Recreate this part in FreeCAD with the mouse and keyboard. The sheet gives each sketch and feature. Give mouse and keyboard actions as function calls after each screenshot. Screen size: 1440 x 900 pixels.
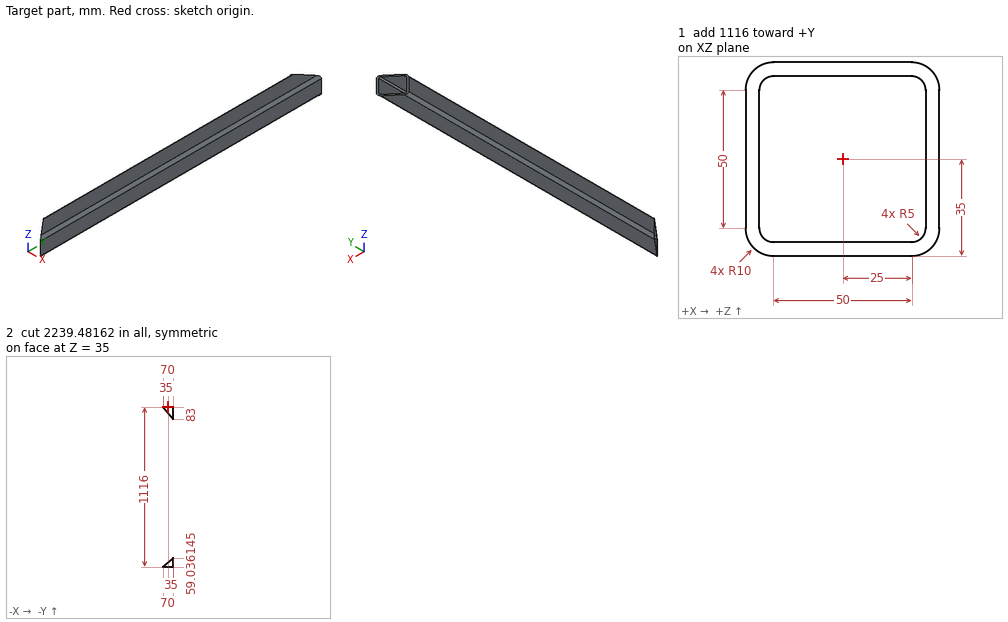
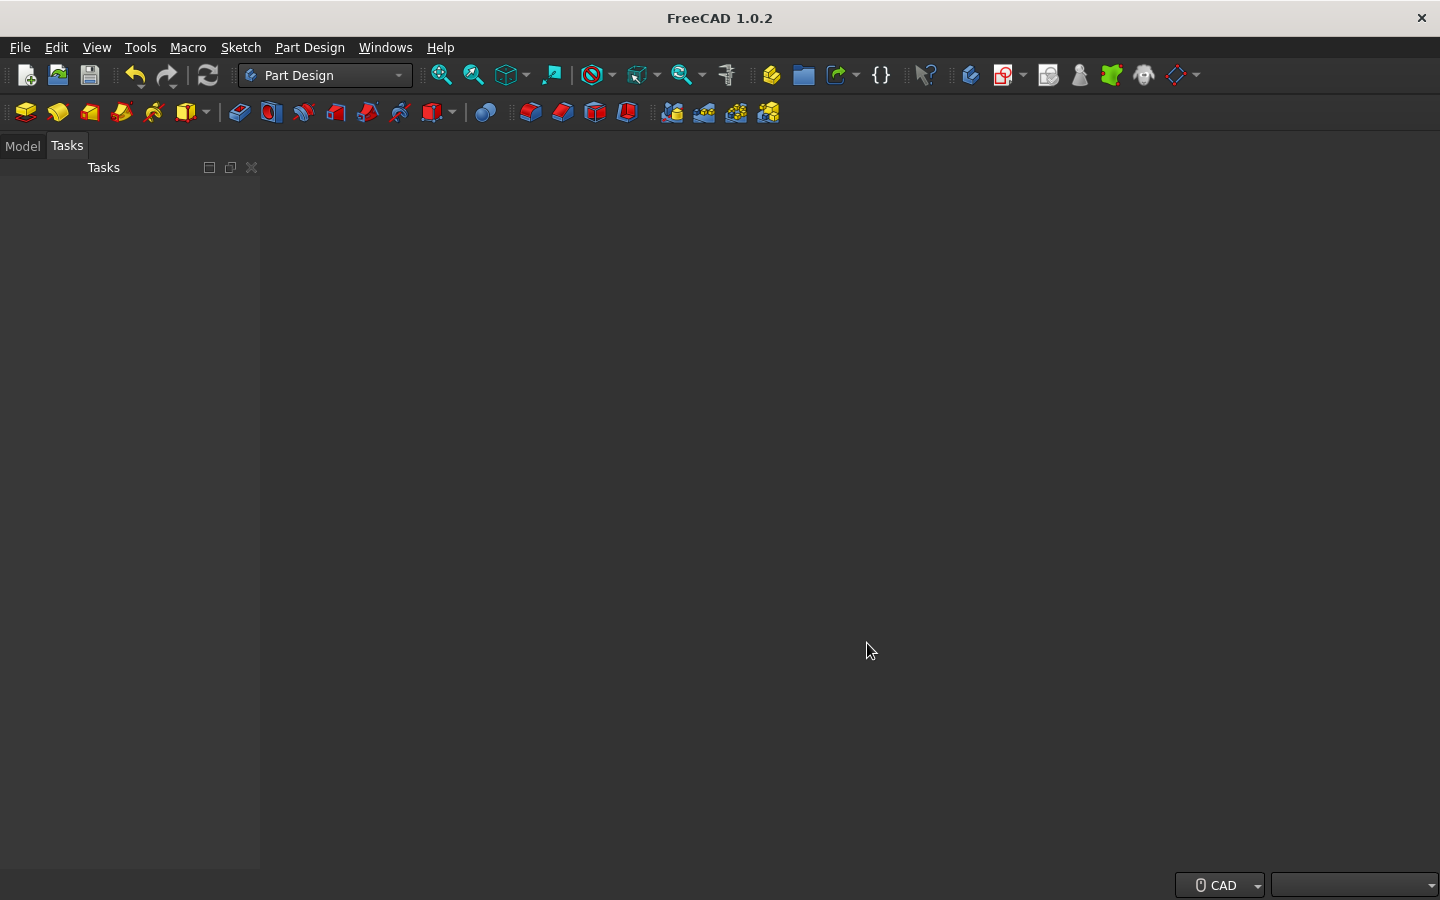
click(26, 76)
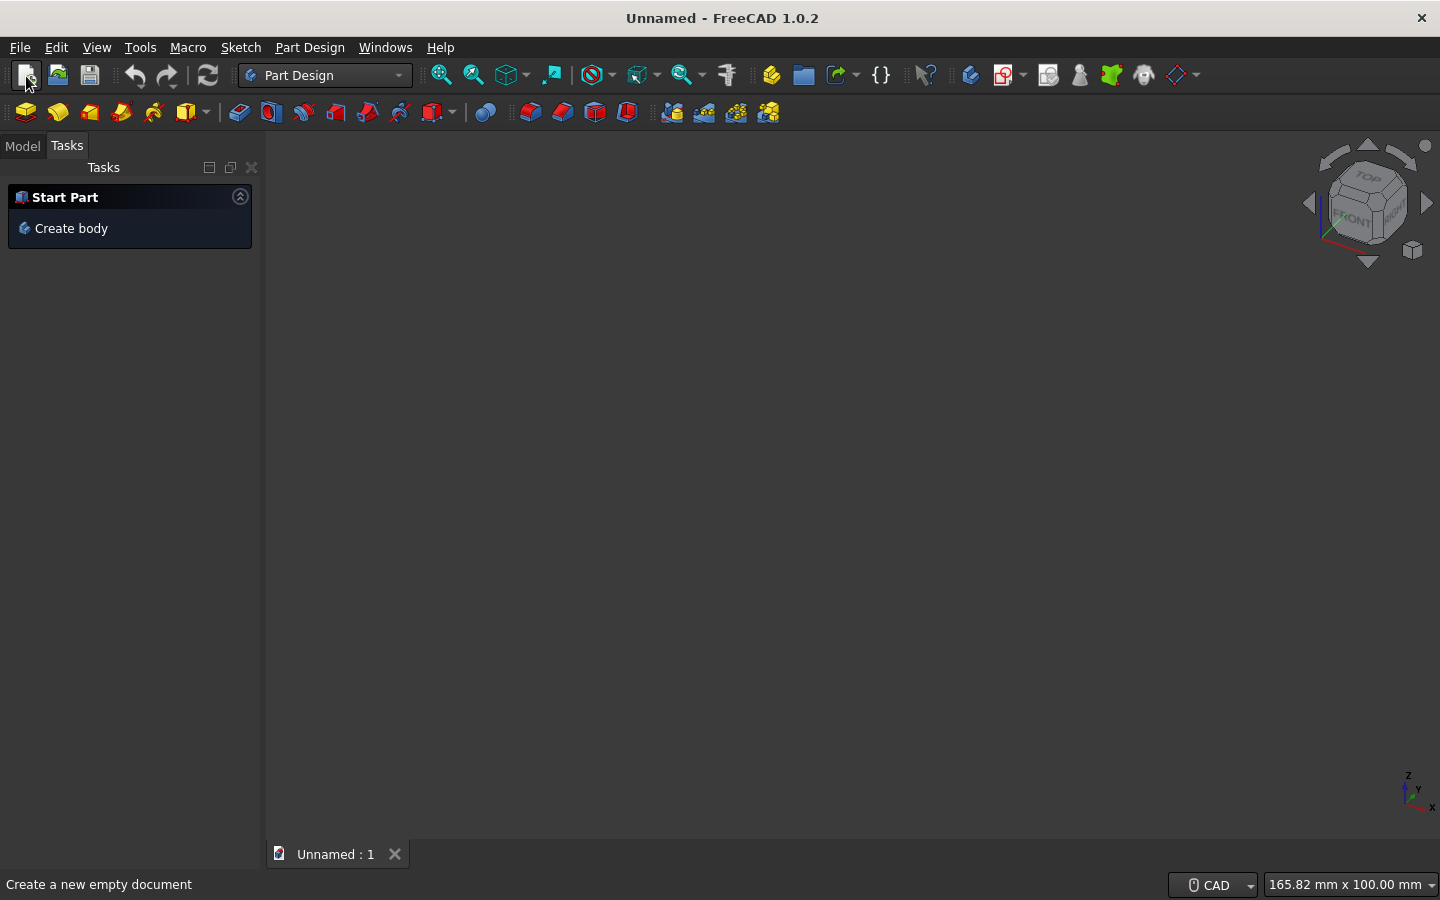
click(1004, 76)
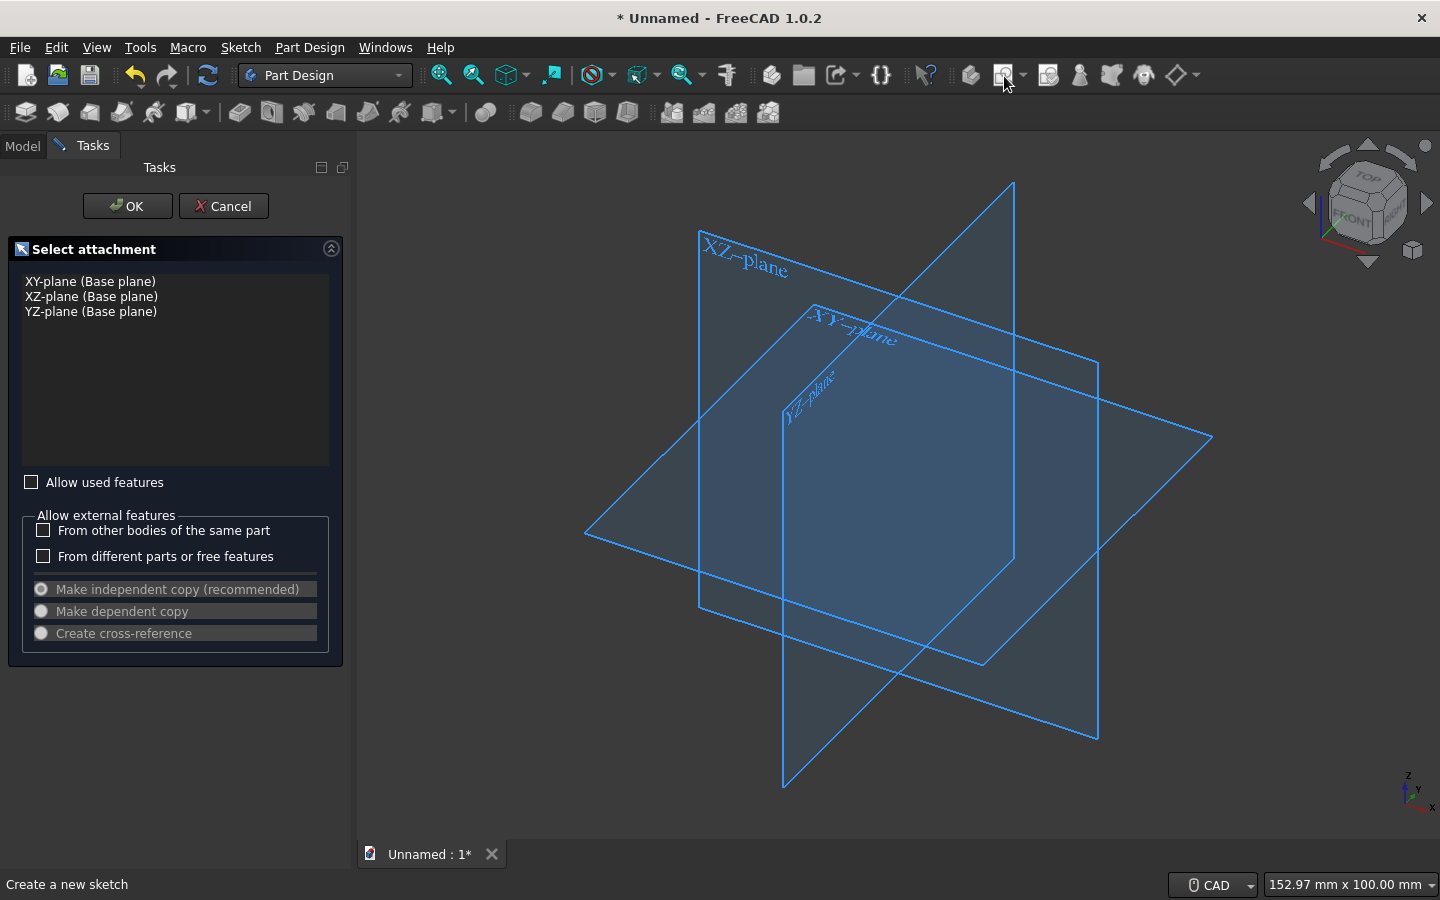
click(82, 296)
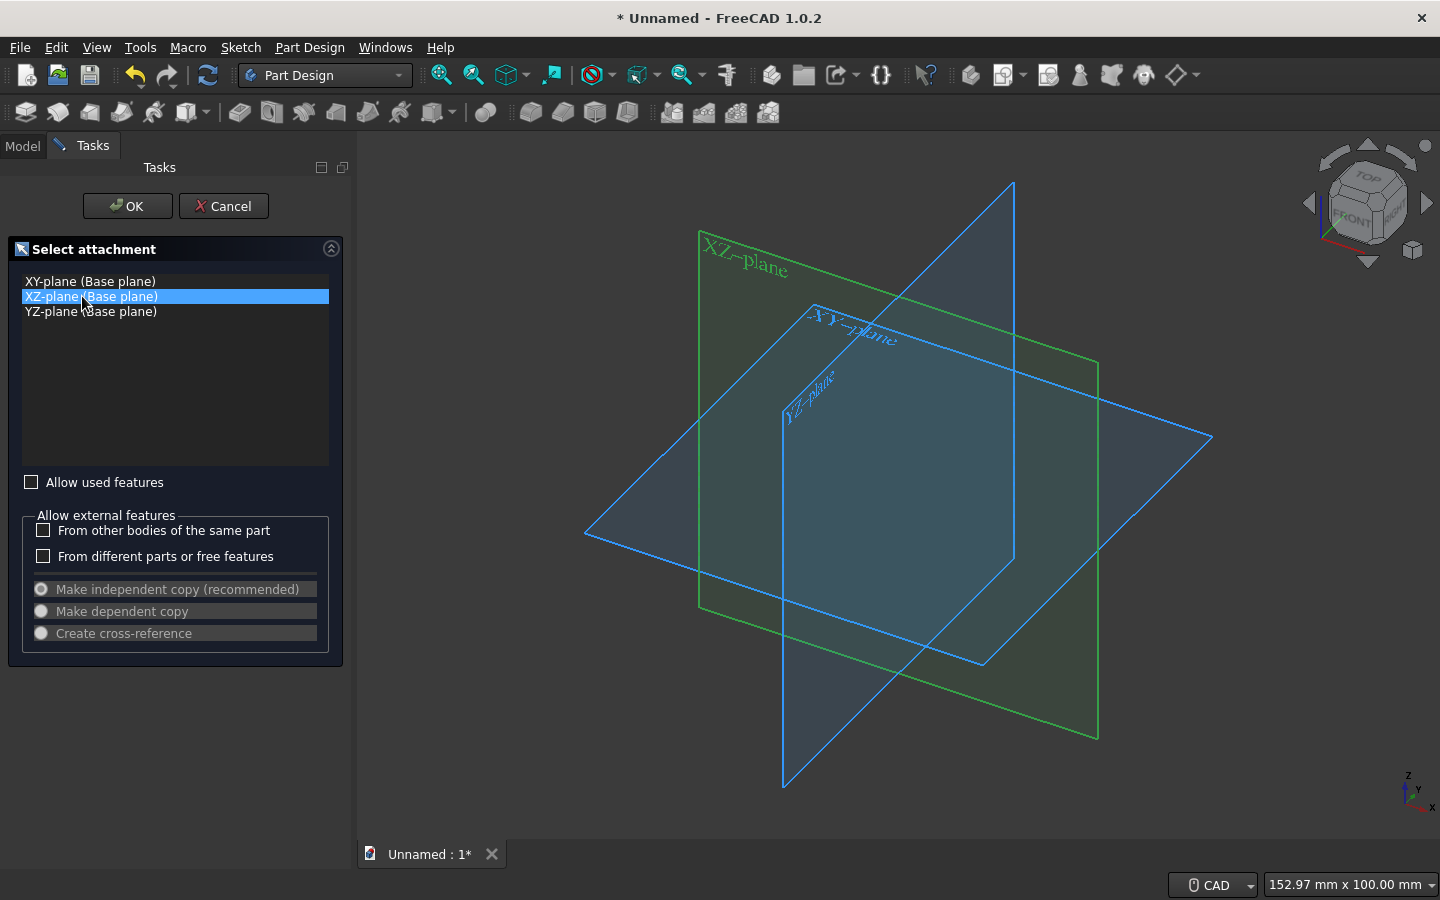
click(128, 206)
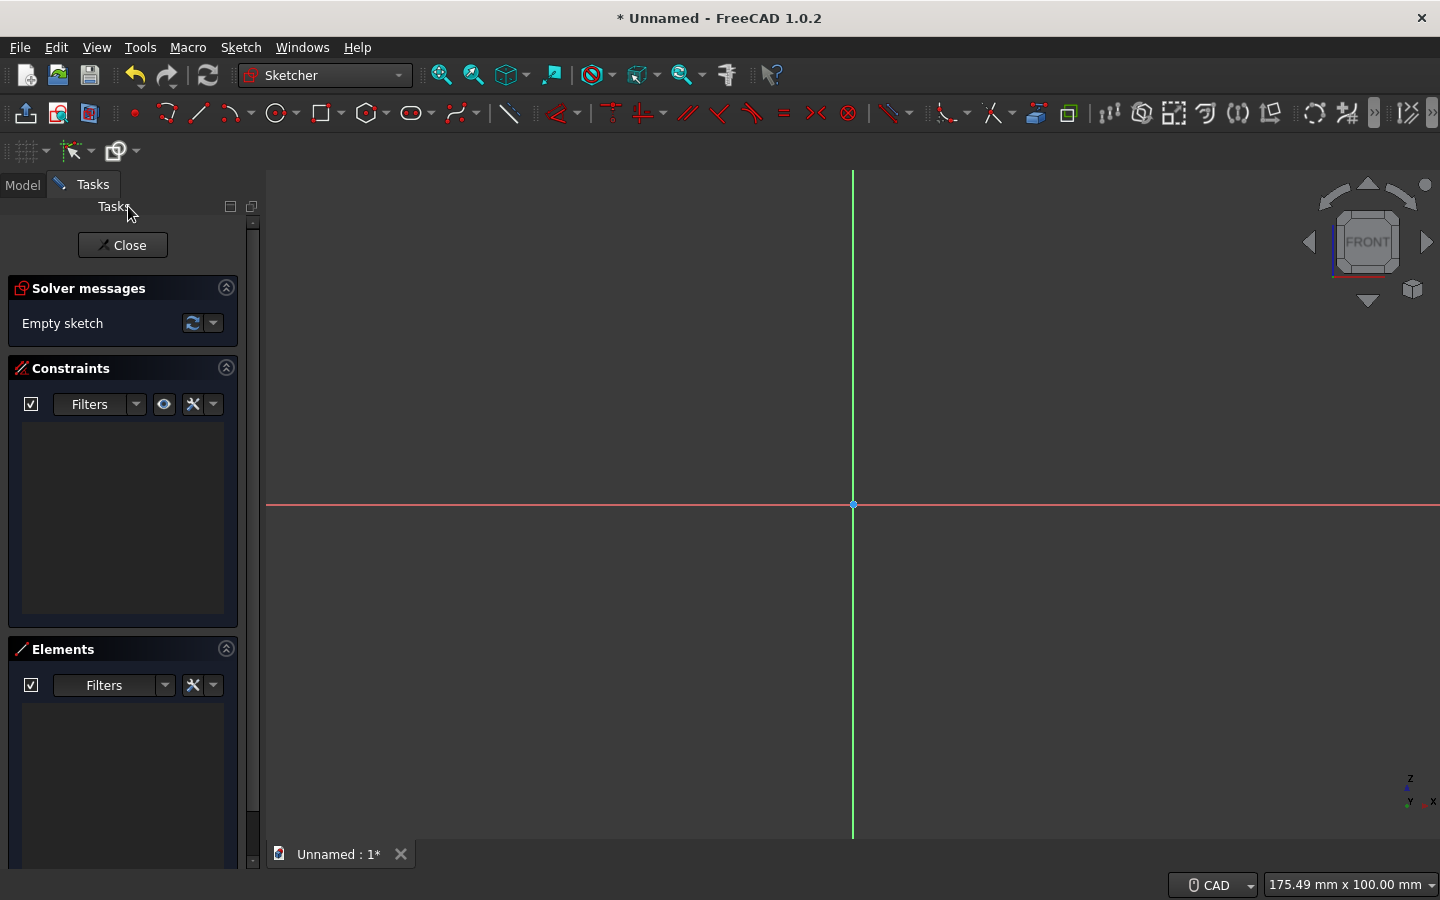
key(g)
key(l)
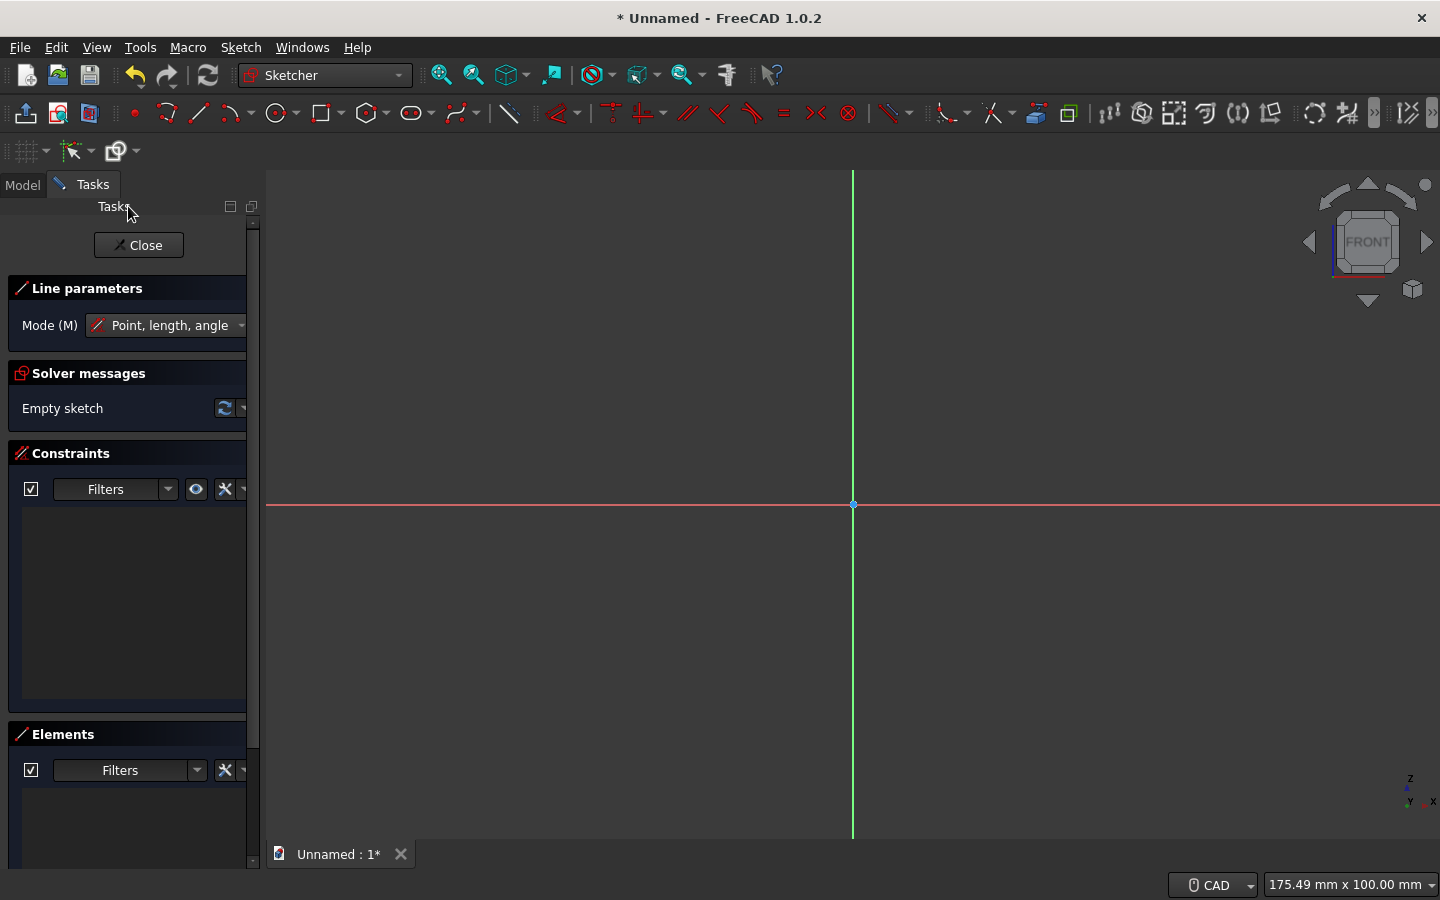
click(1020, 739)
click(686, 739)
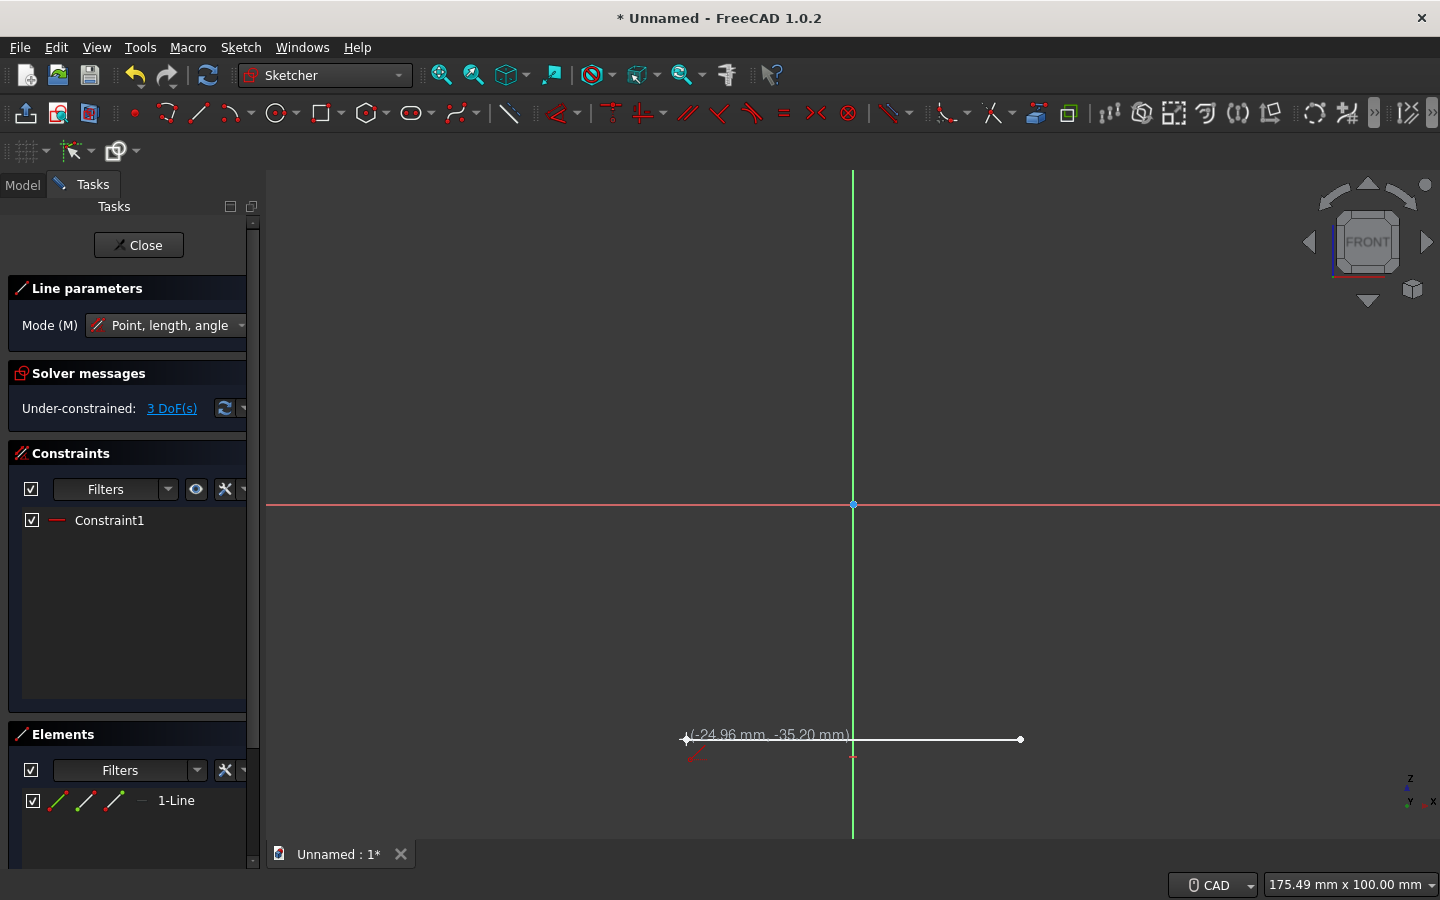
click(619, 672)
click(619, 337)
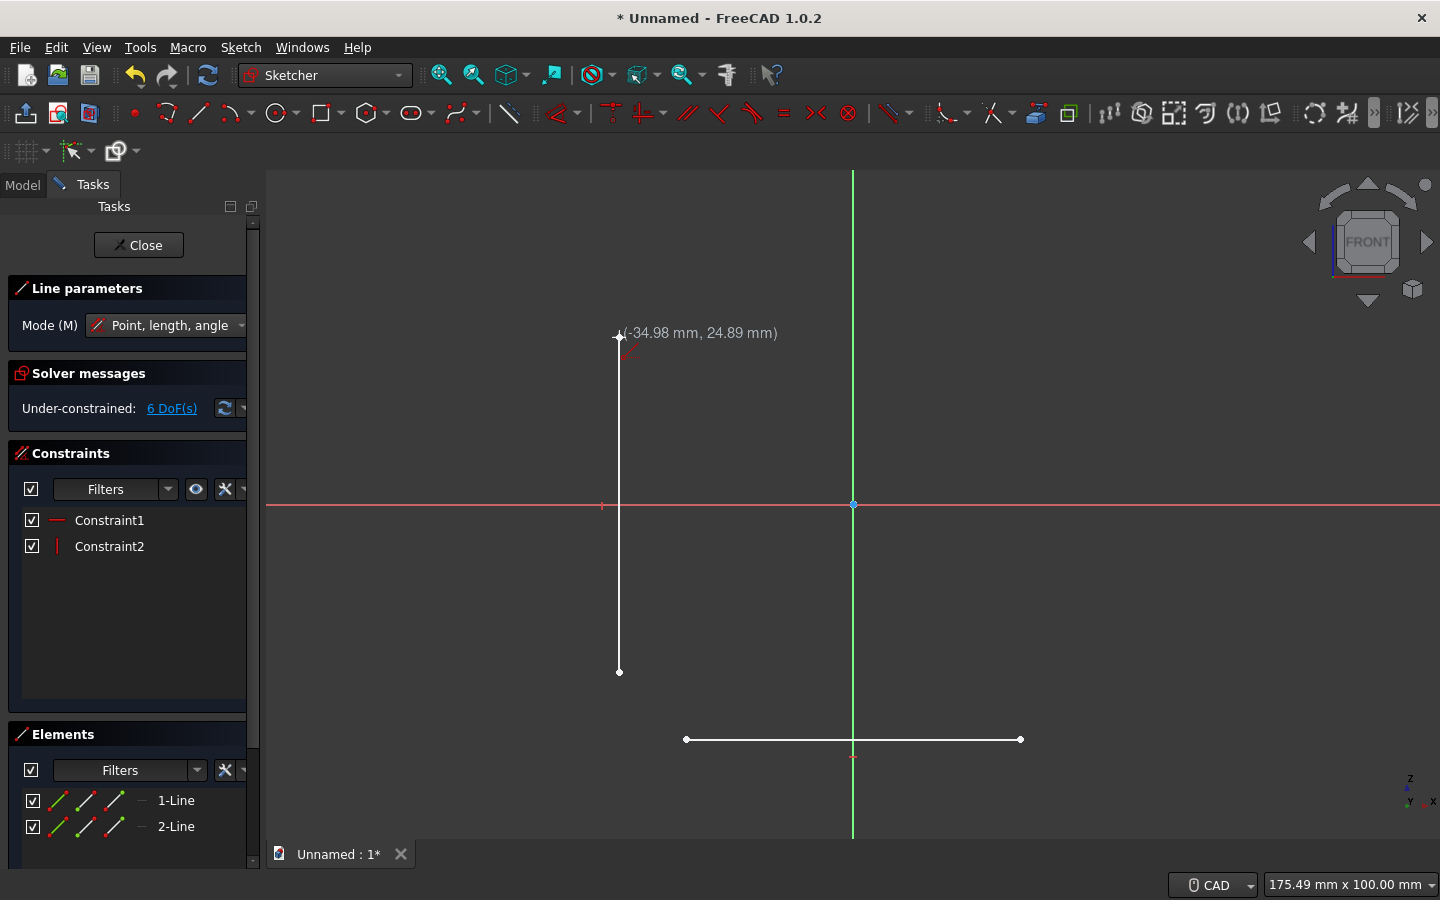
click(686, 270)
click(1020, 270)